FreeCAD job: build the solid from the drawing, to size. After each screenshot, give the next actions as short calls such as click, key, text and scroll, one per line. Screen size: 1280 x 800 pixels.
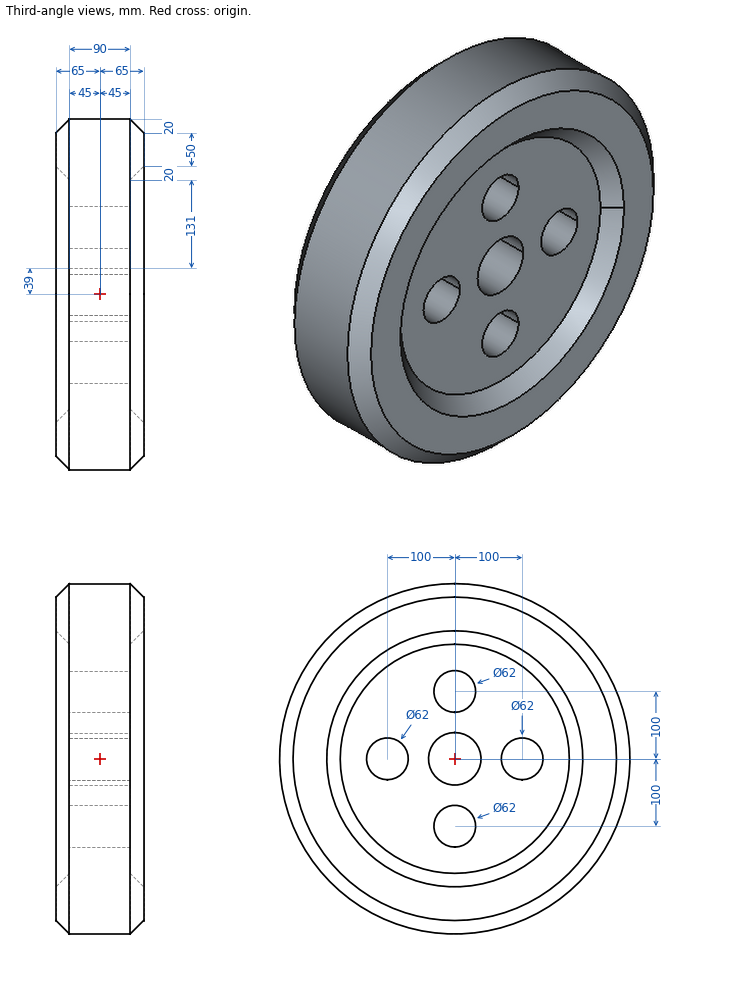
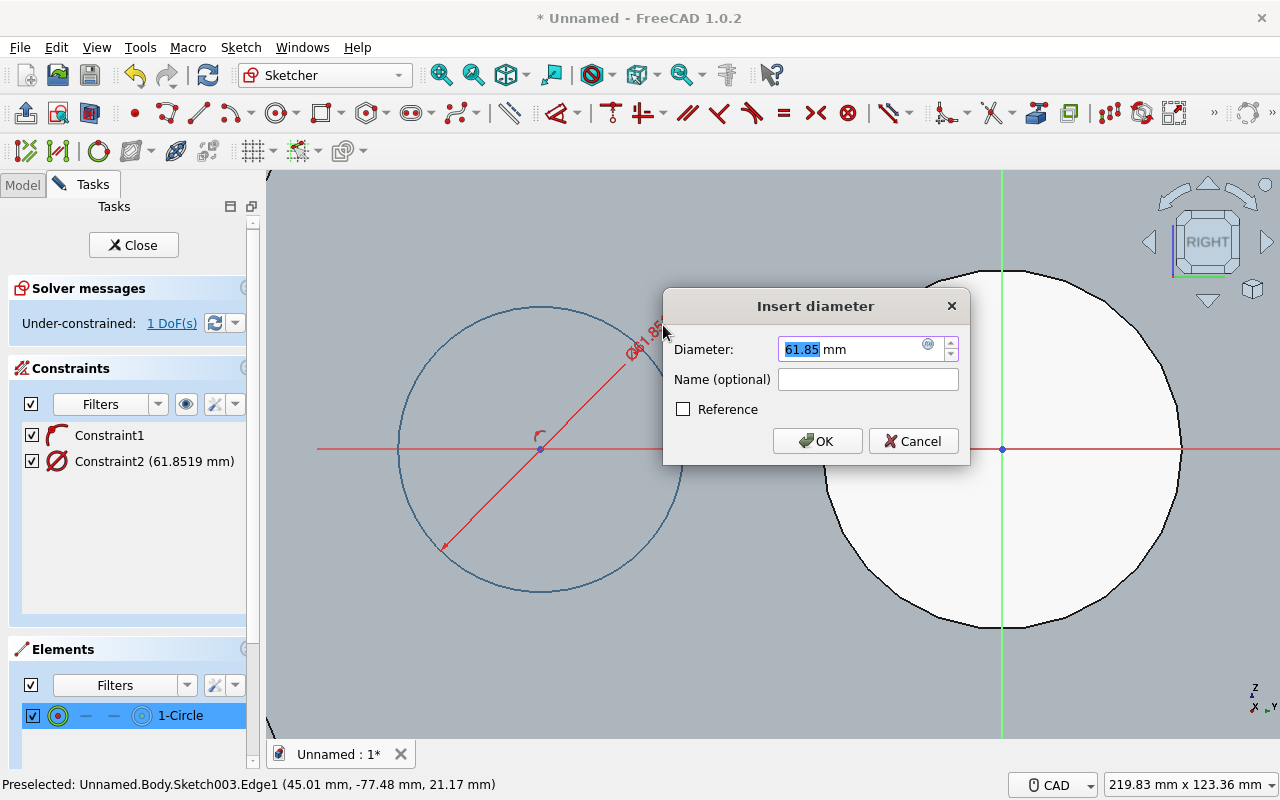
text(62)
key(Return)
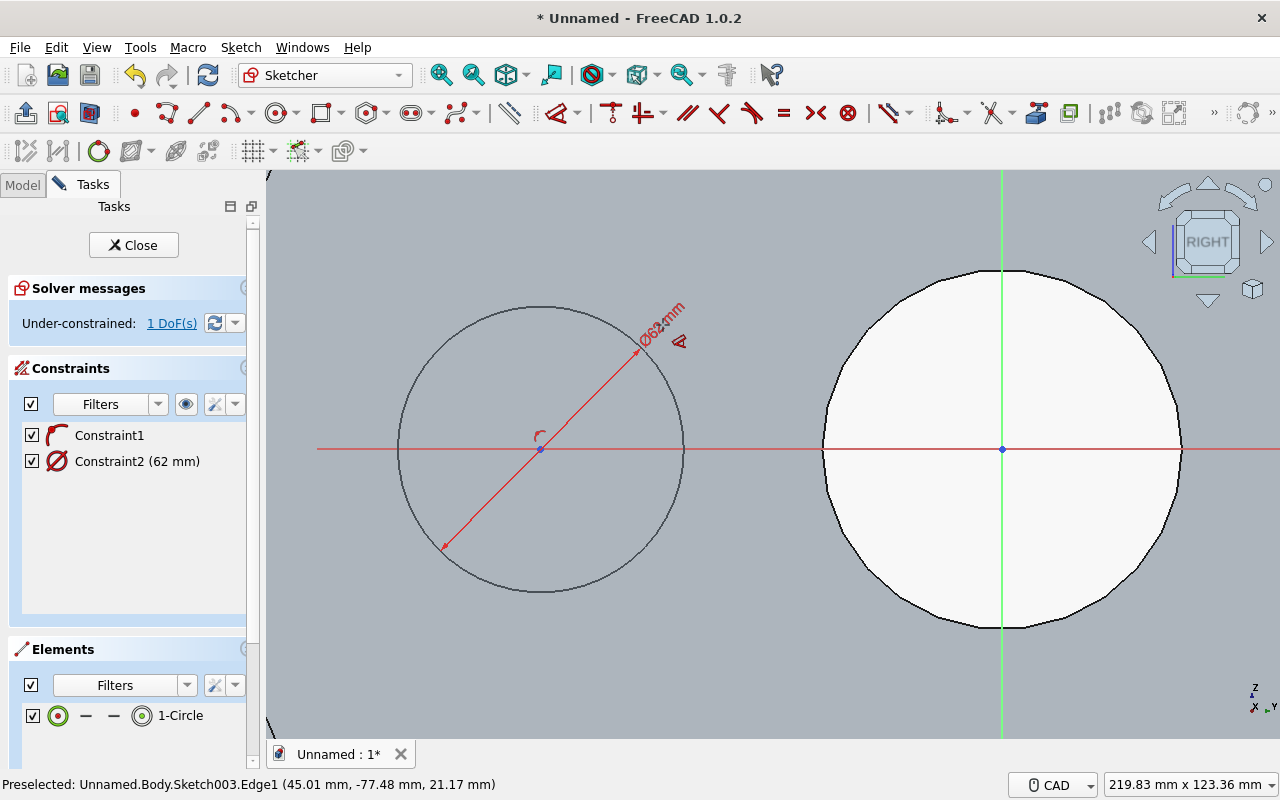
click(541, 449)
click(771, 483)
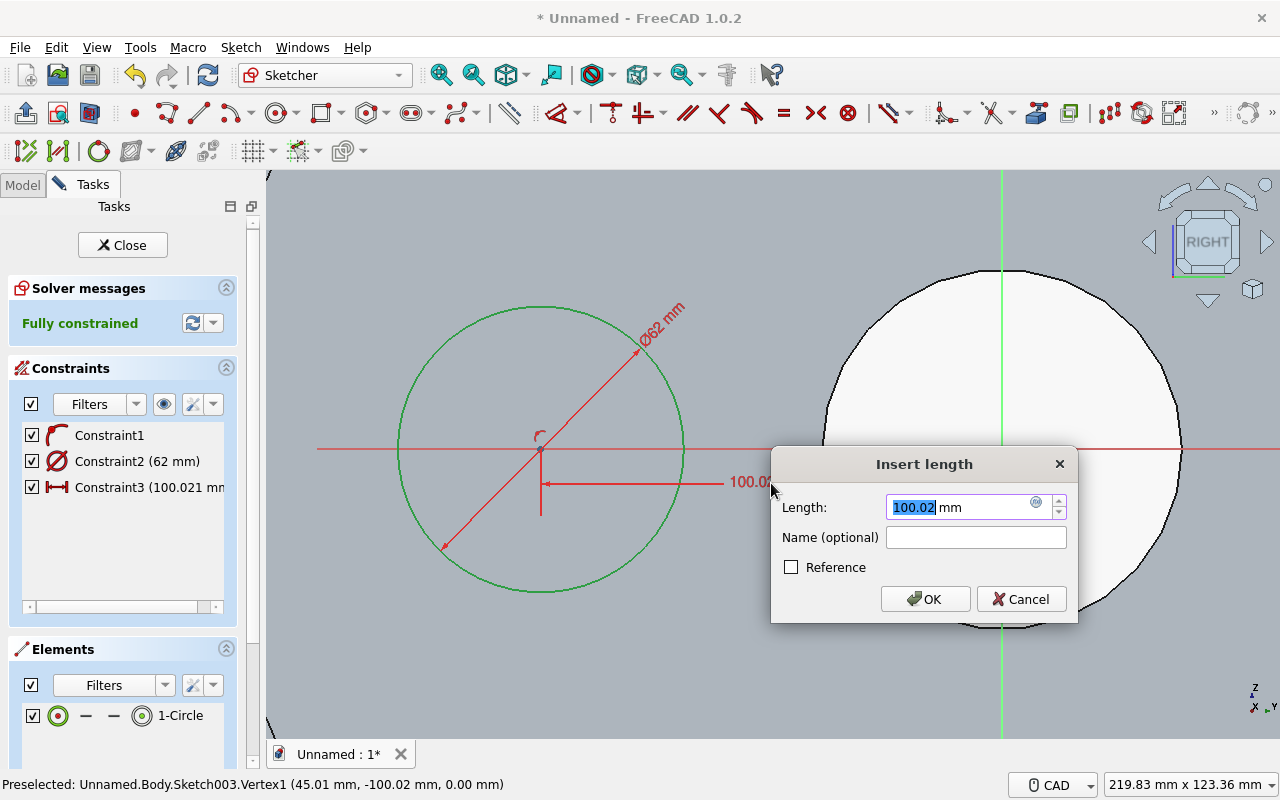
text(100)
key(Return)
key(Escape)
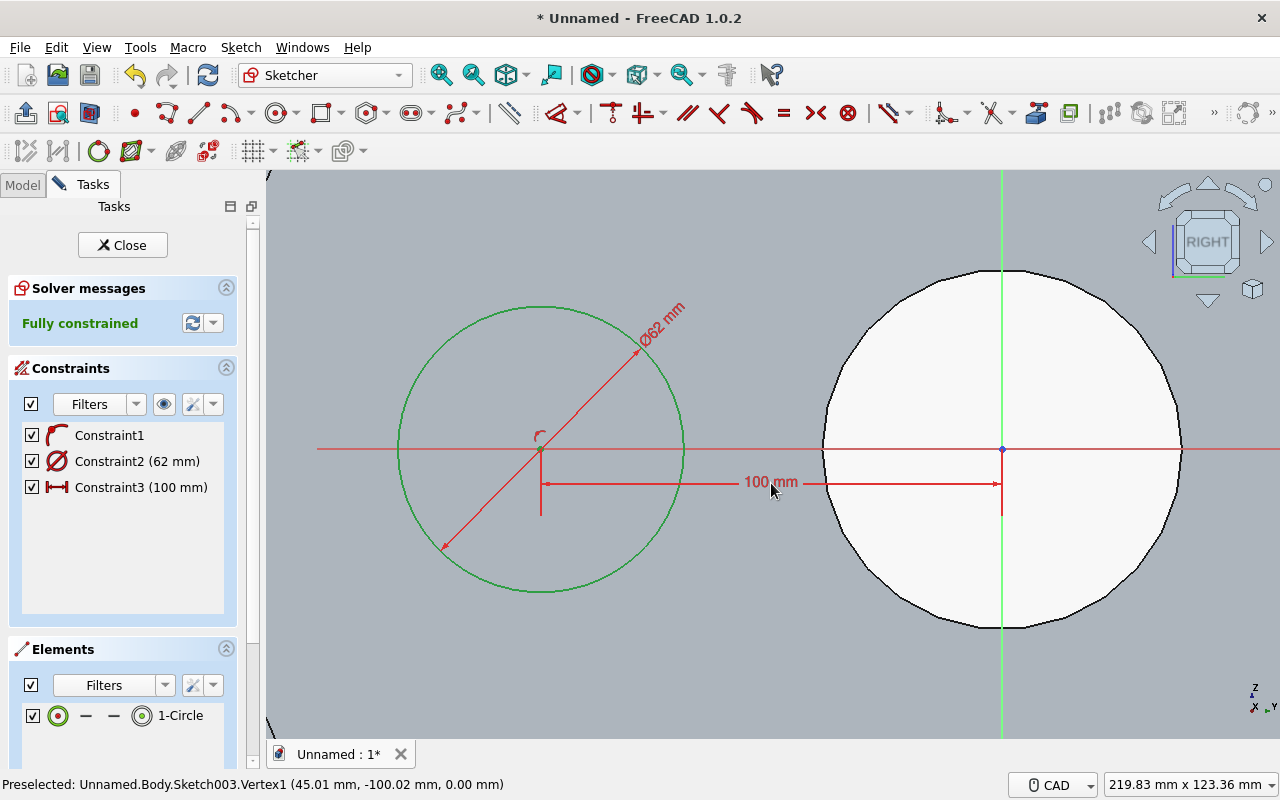
click(123, 245)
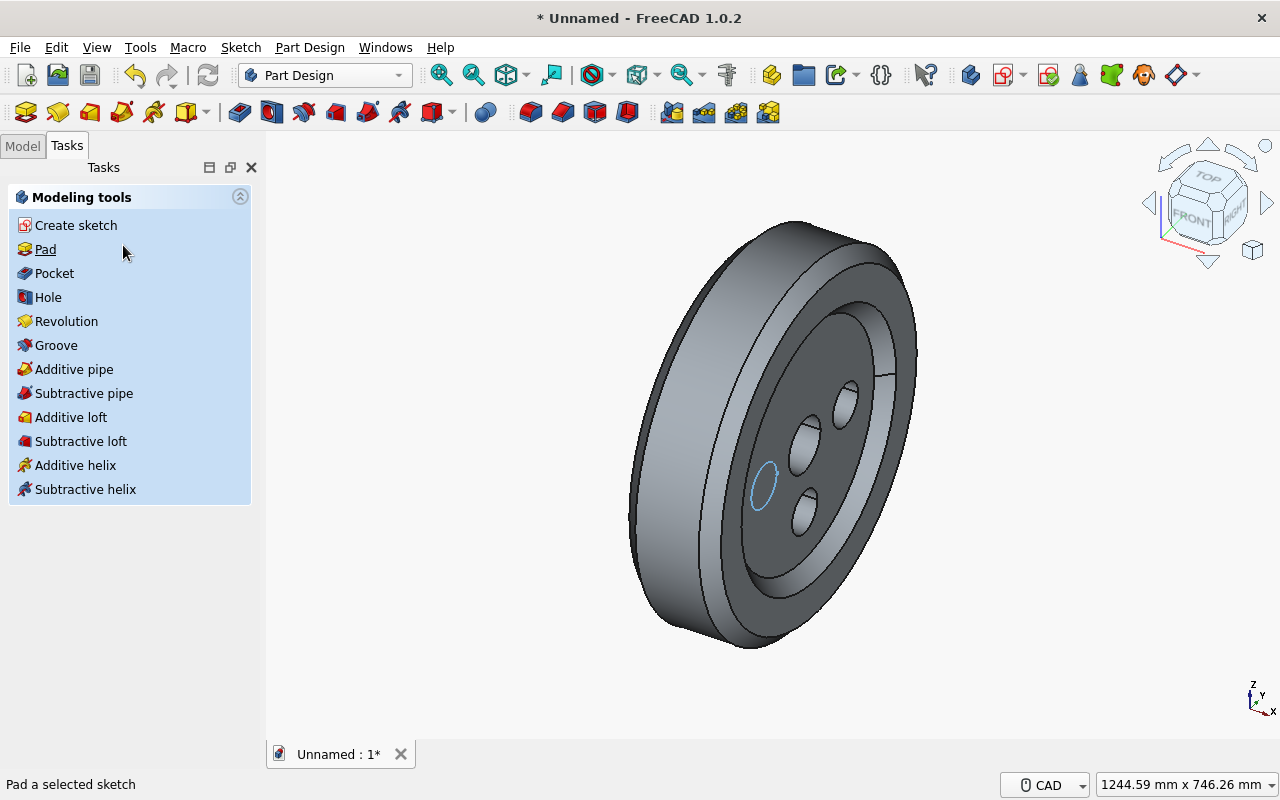
click(240, 112)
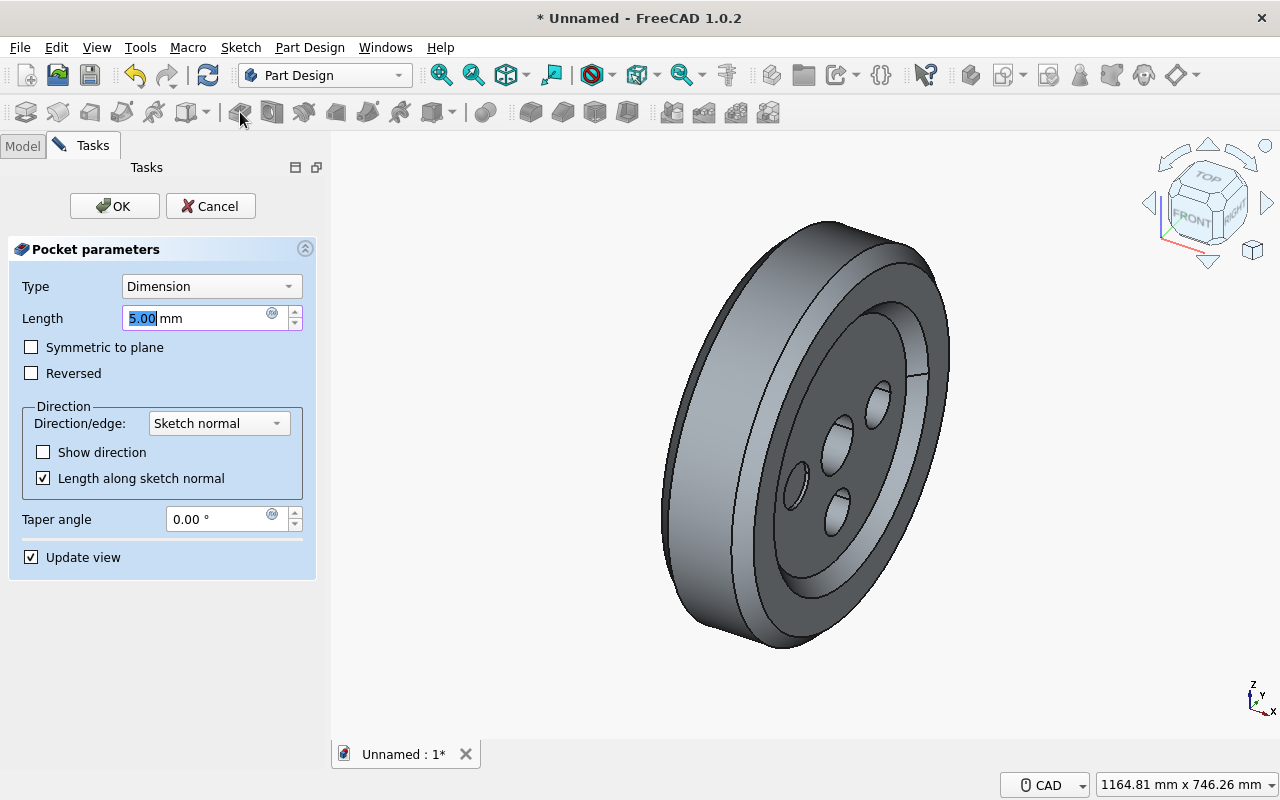
click(212, 286)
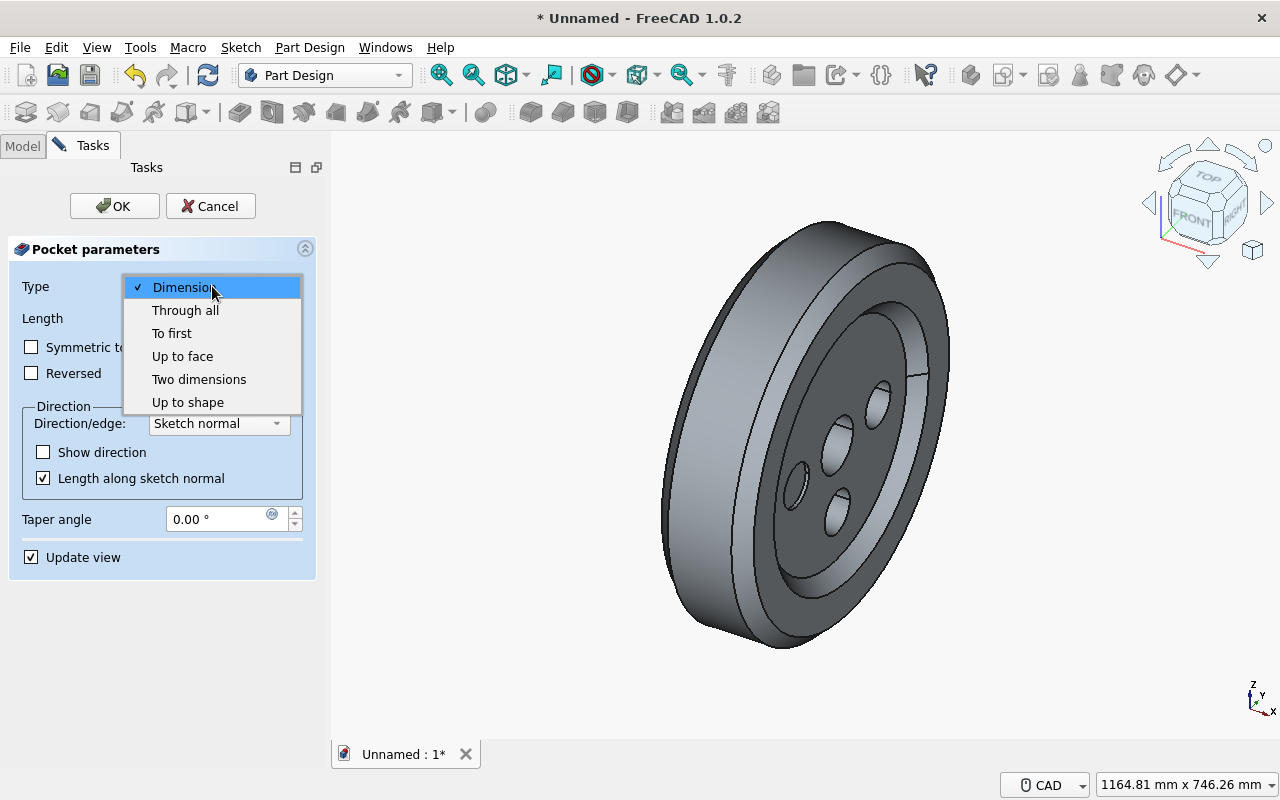
click(212, 334)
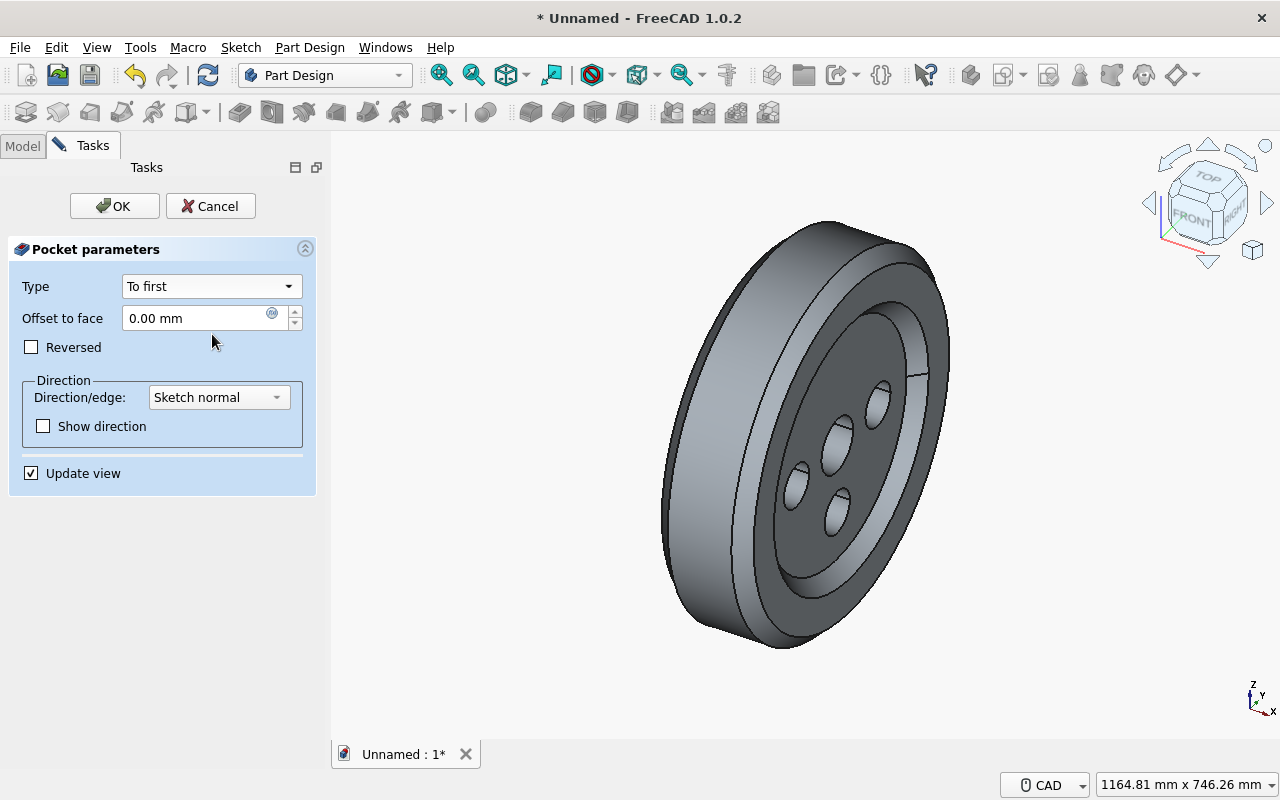
click(115, 206)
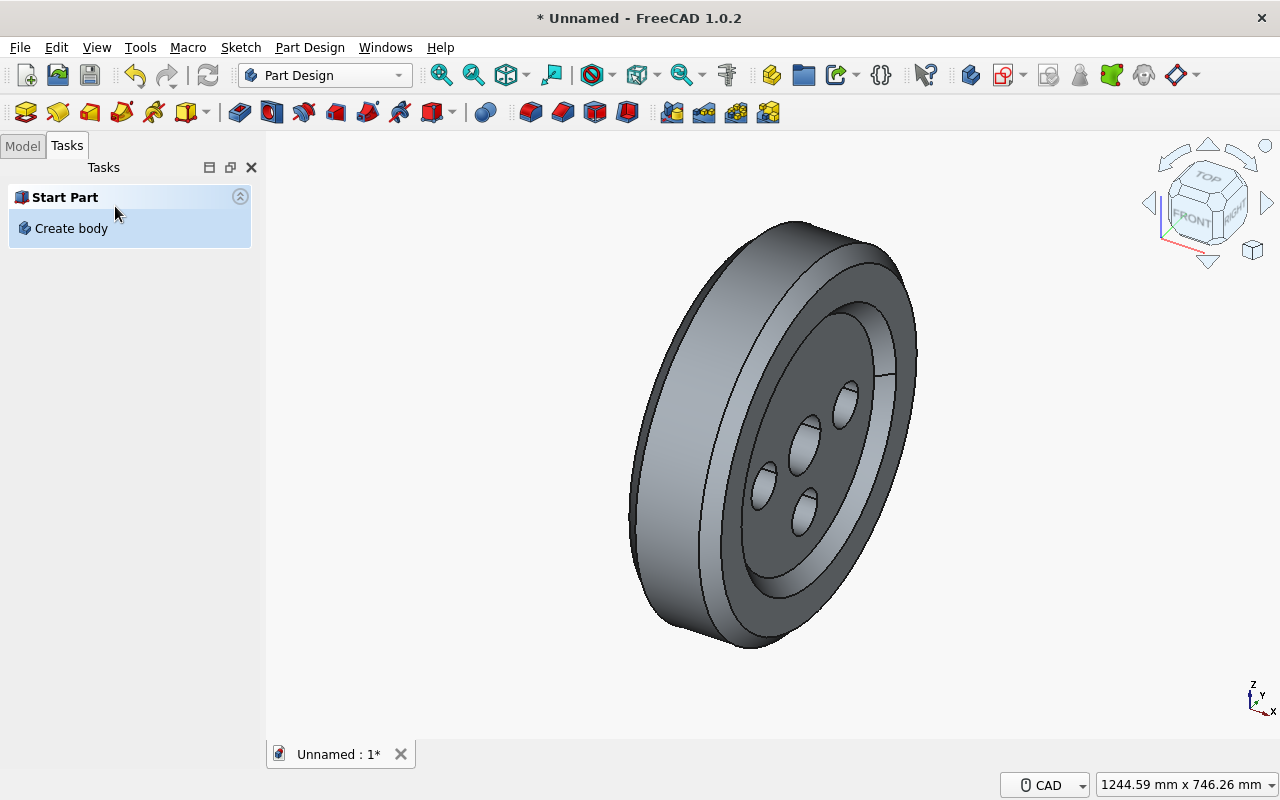
click(825, 360)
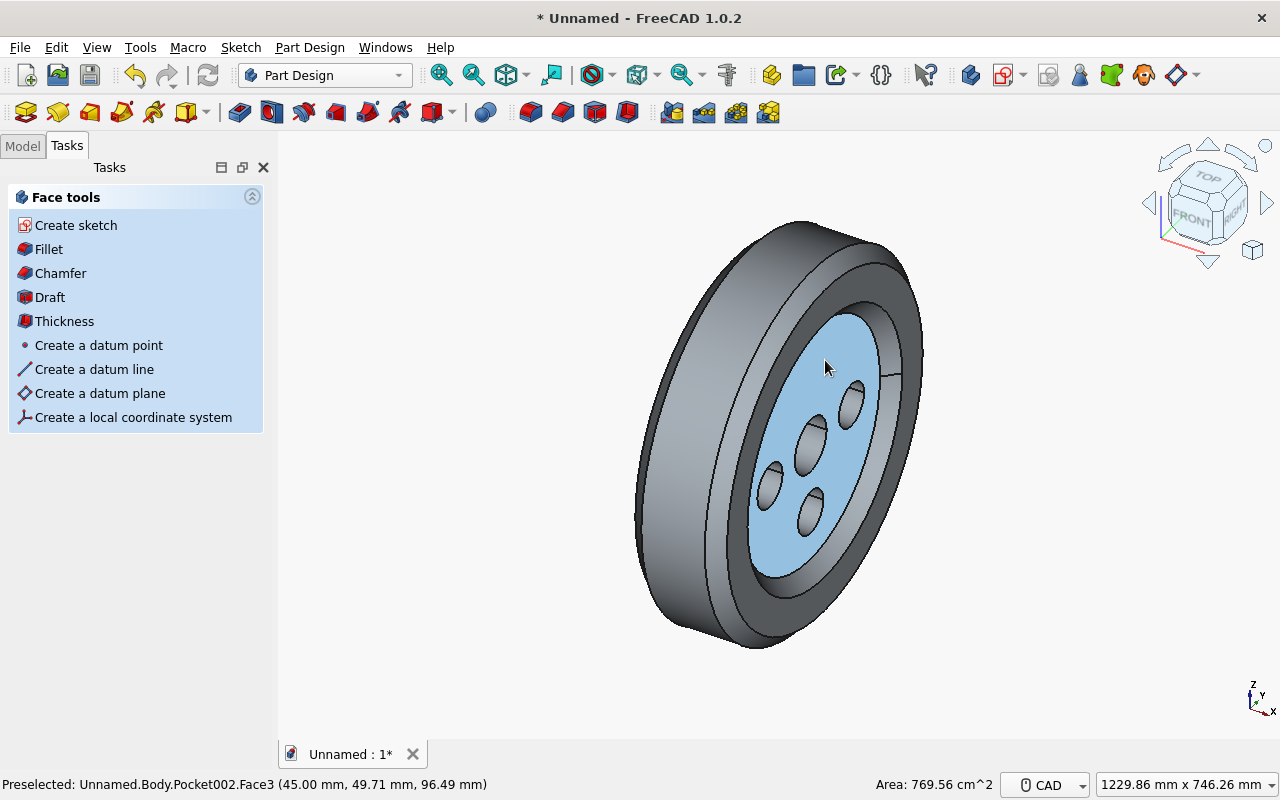
click(1004, 76)